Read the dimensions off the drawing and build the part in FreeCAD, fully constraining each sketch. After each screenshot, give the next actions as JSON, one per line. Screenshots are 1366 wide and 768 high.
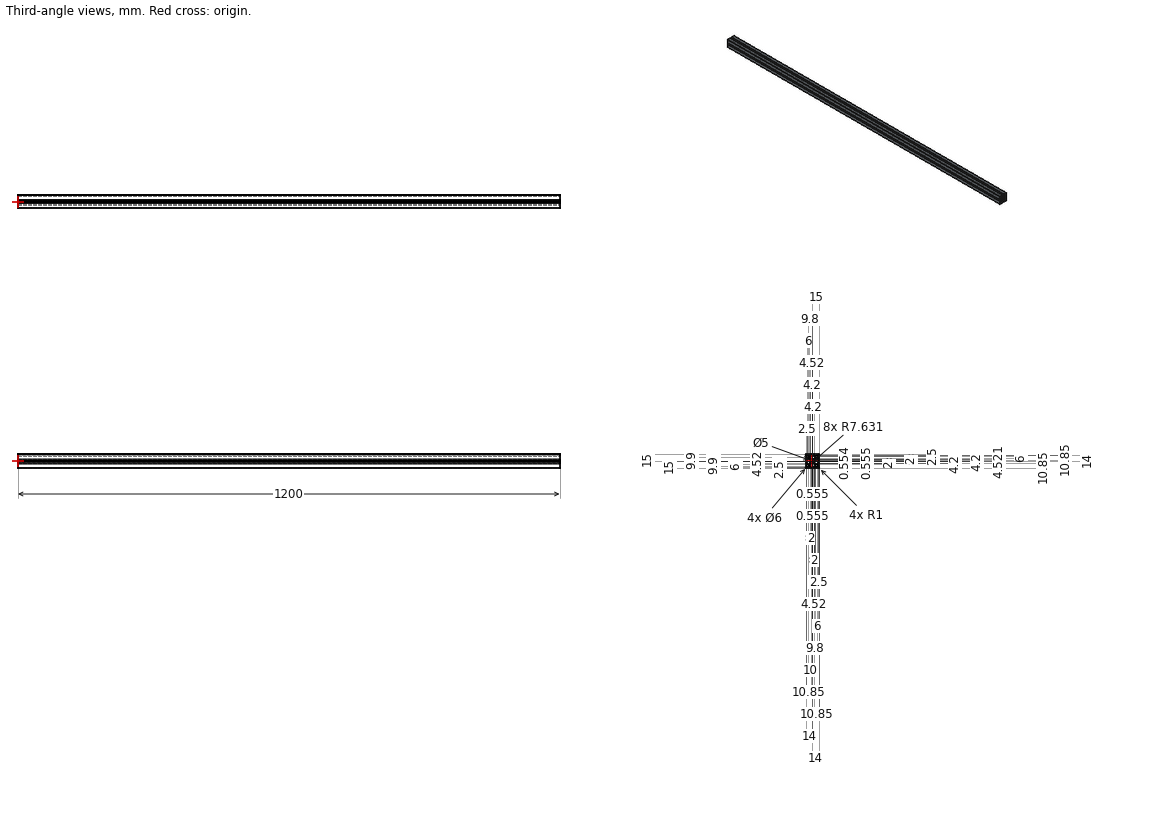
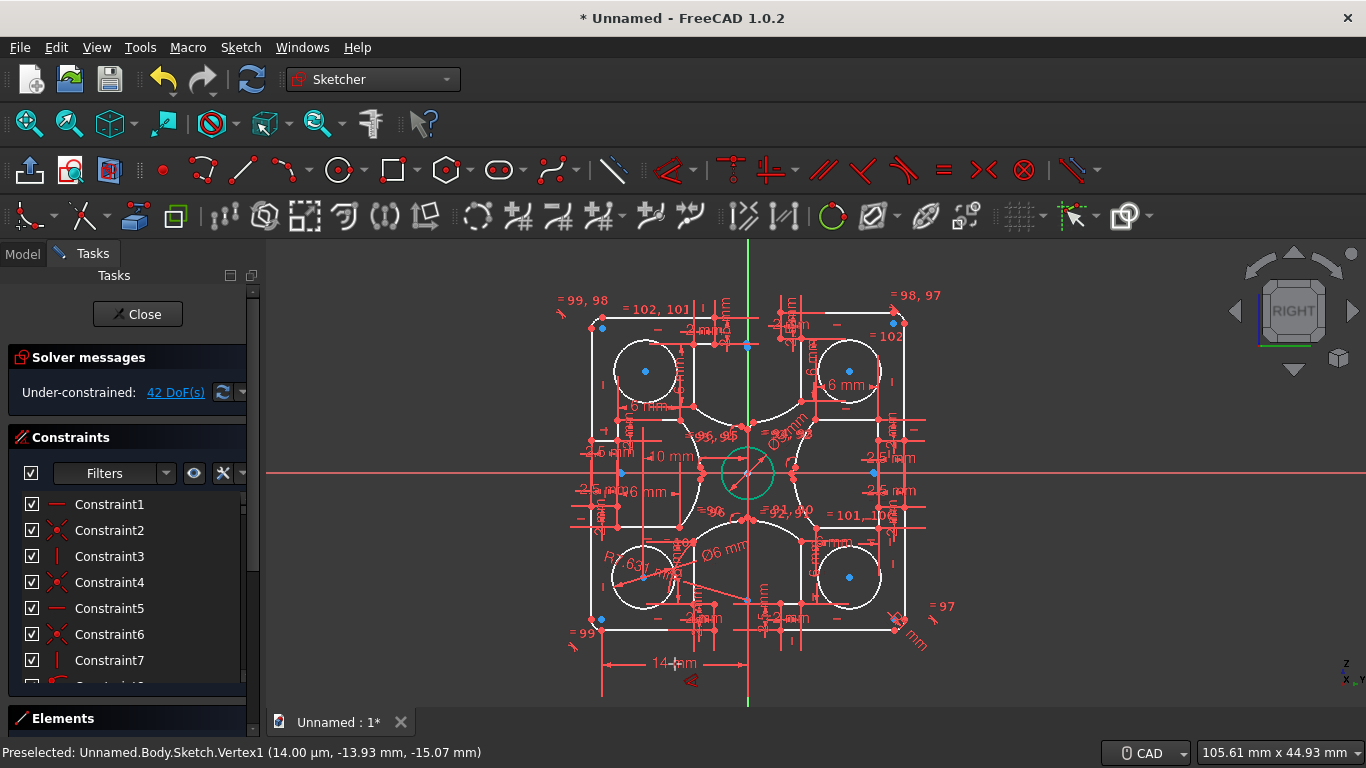
{"action": "left_click", "coordinate": [602, 630]}
{"action": "left_click", "coordinate": [568, 552]}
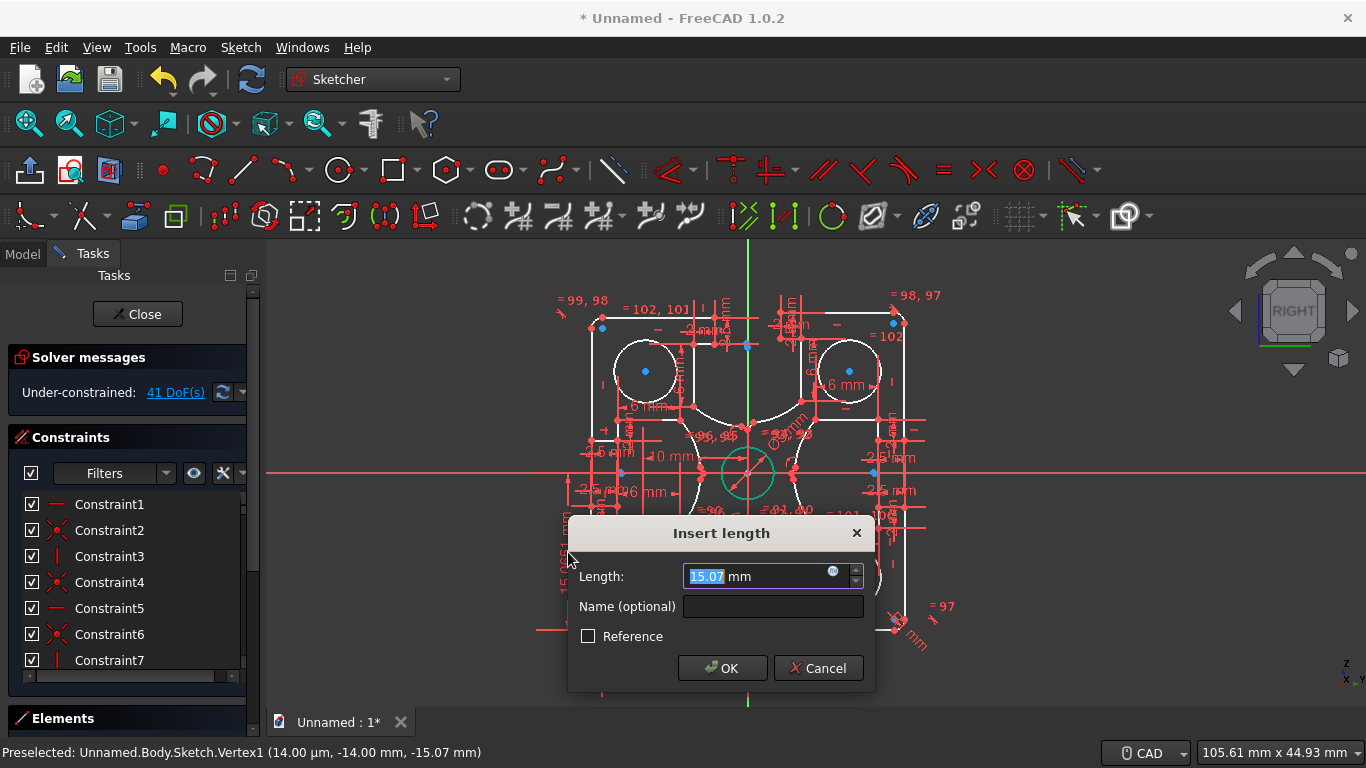
{"action": "type", "text": "15"}
{"action": "key", "text": "Return"}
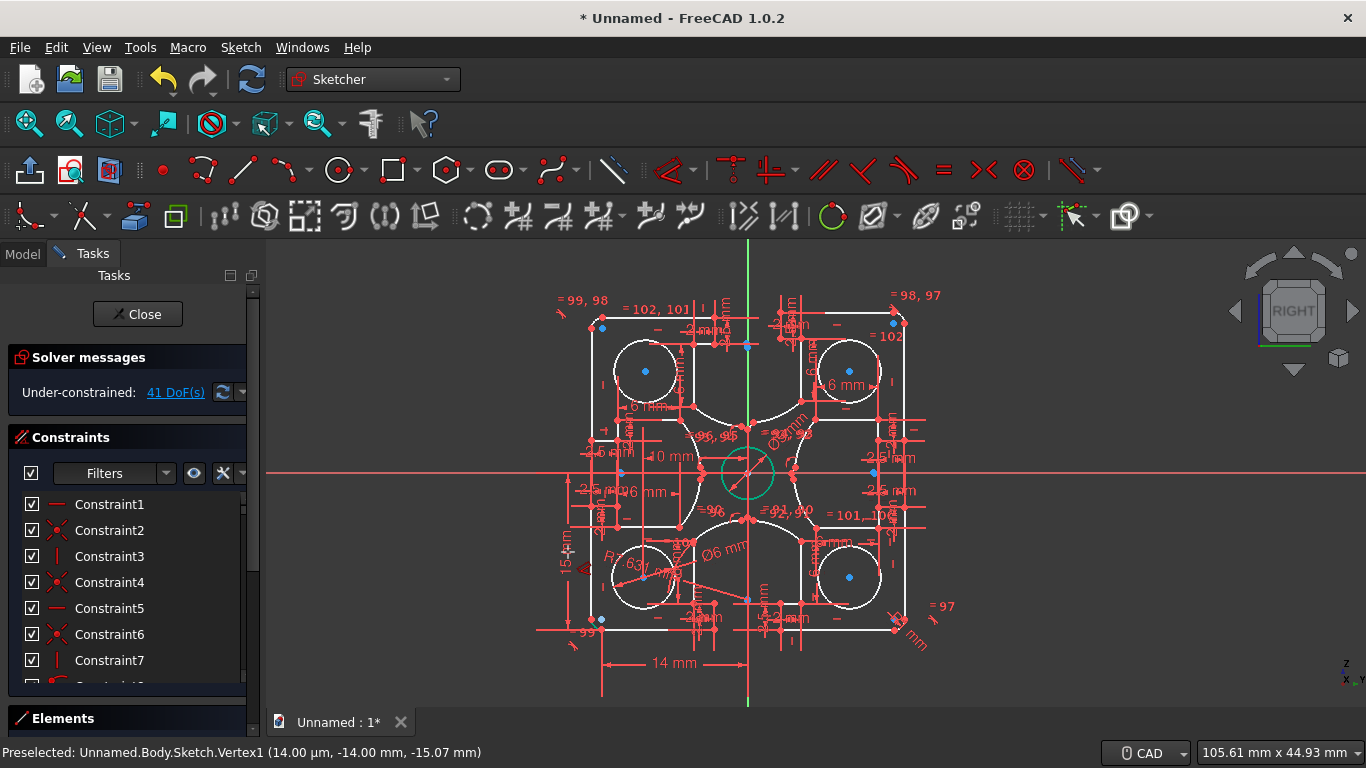
{"action": "left_click", "coordinate": [781, 630]}
{"action": "left_click", "coordinate": [815, 497]}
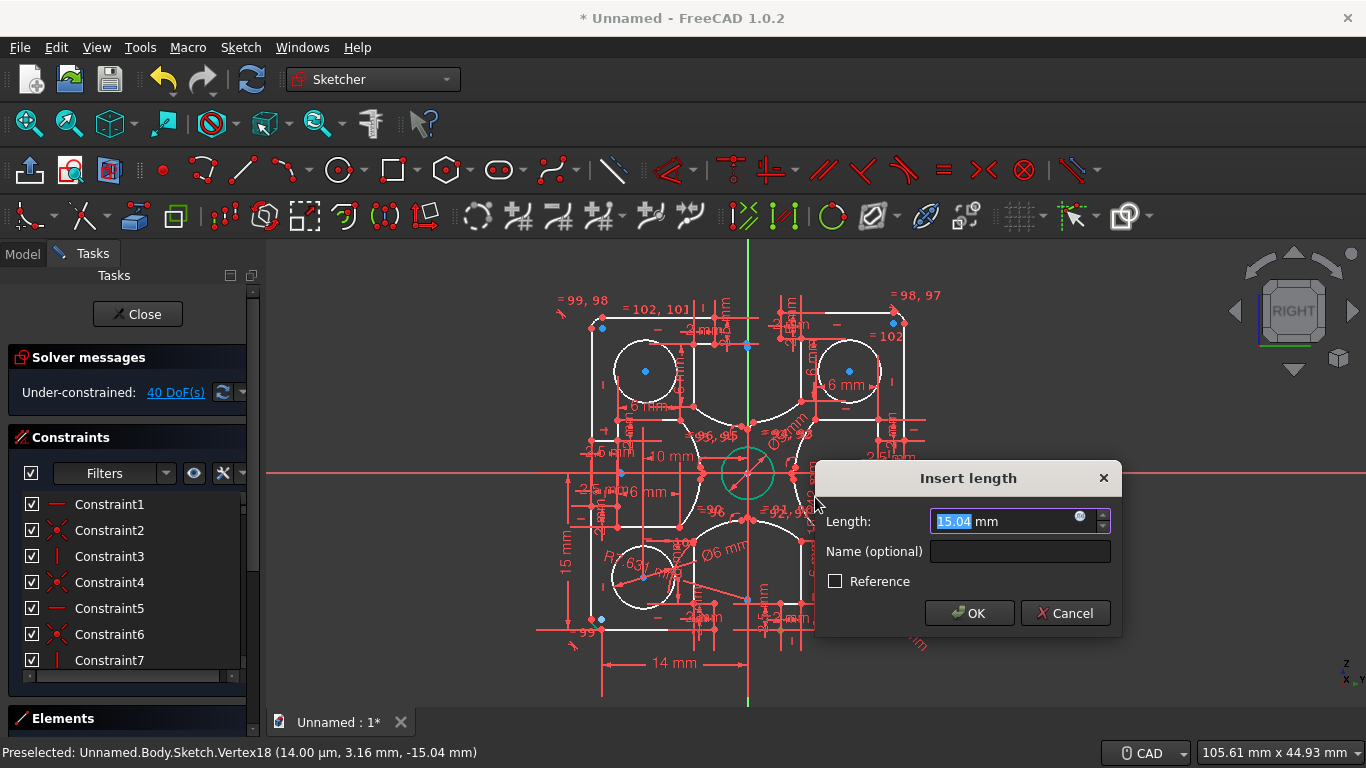
{"action": "type", "text": "15"}
{"action": "key", "text": "Return"}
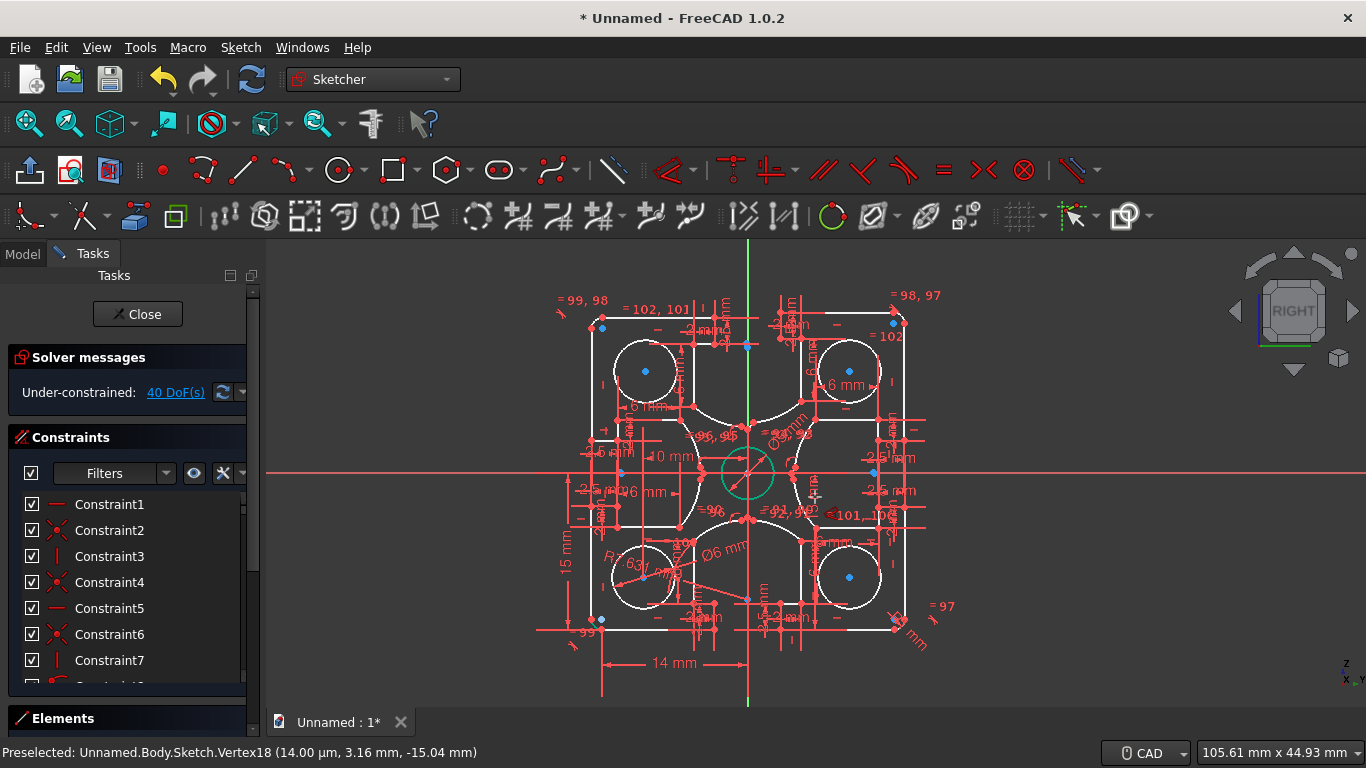
{"action": "left_click", "coordinate": [895, 630]}
{"action": "left_click", "coordinate": [821, 664]}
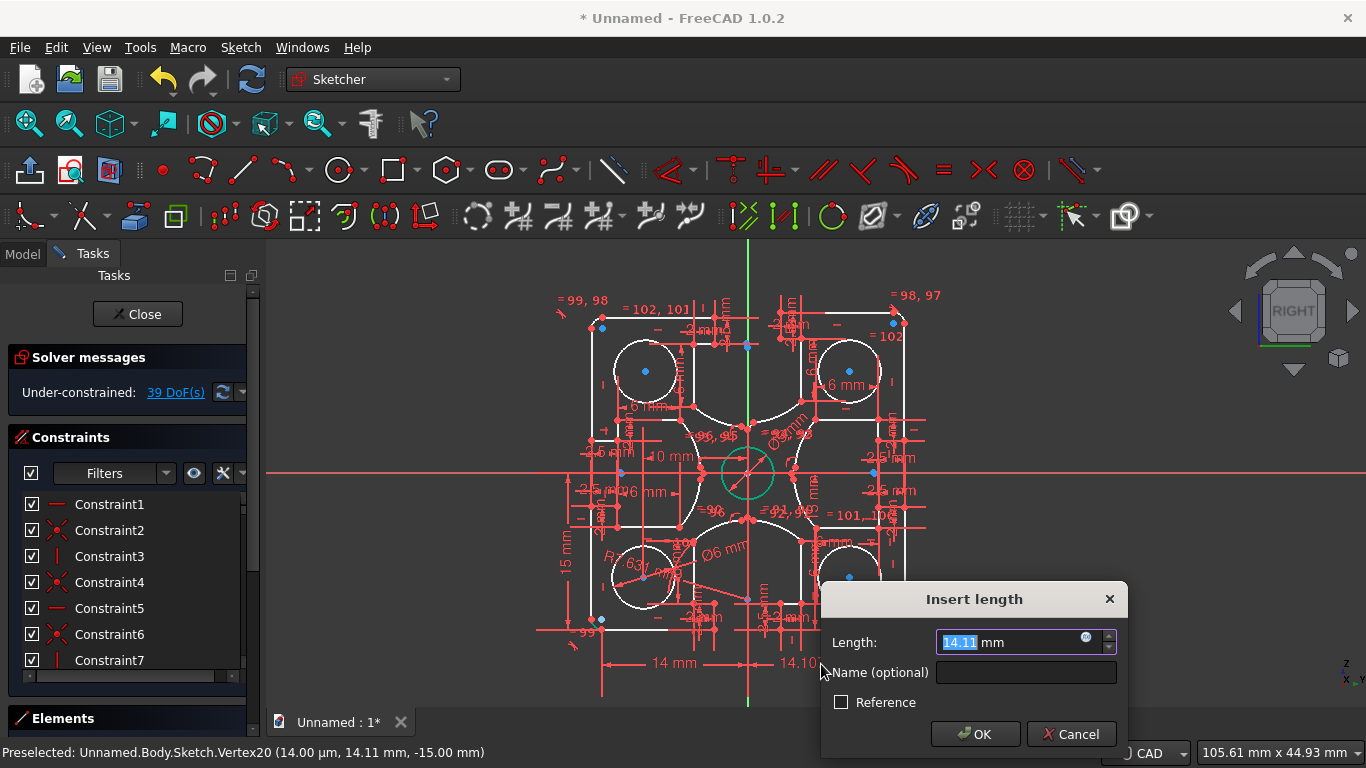
{"action": "type", "text": "14"}
{"action": "key", "text": "Return"}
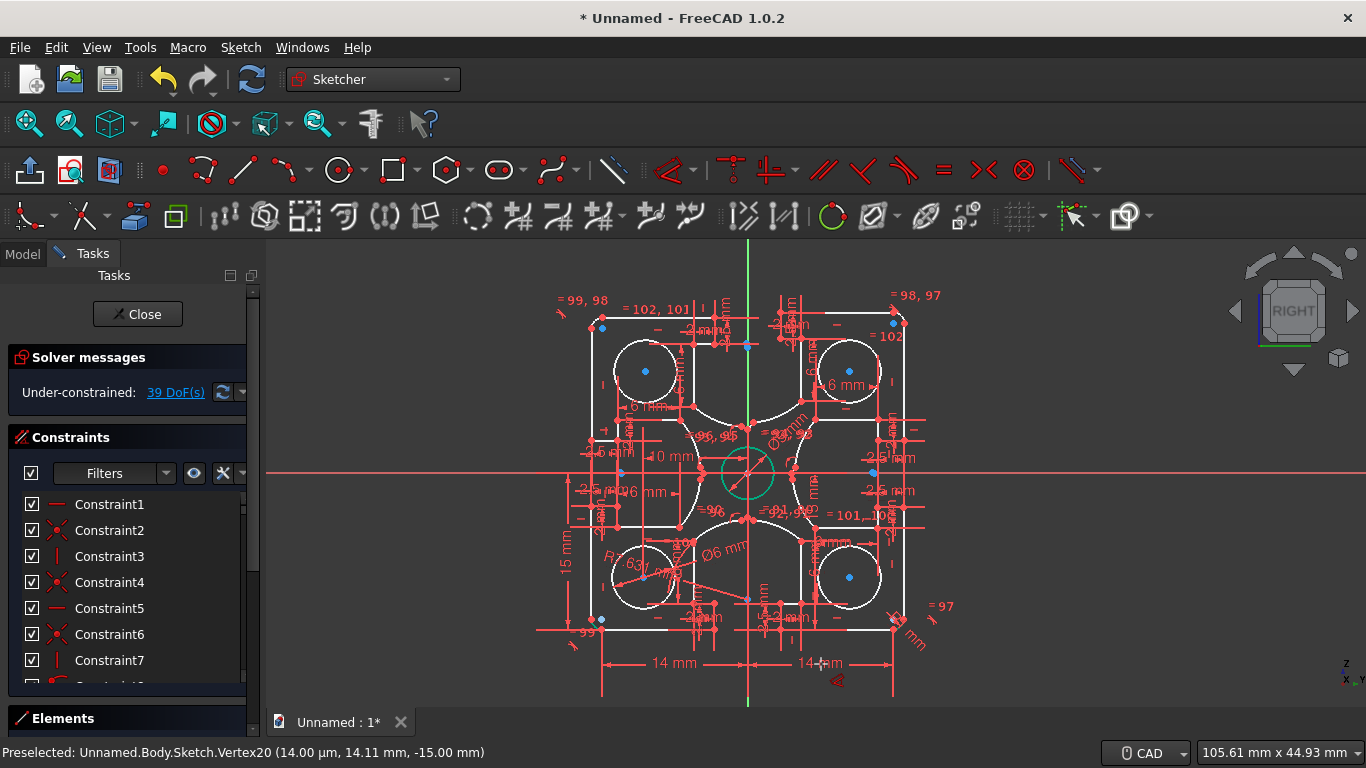
{"action": "left_click", "coordinate": [904, 441]}
{"action": "left_click", "coordinate": [881, 407]}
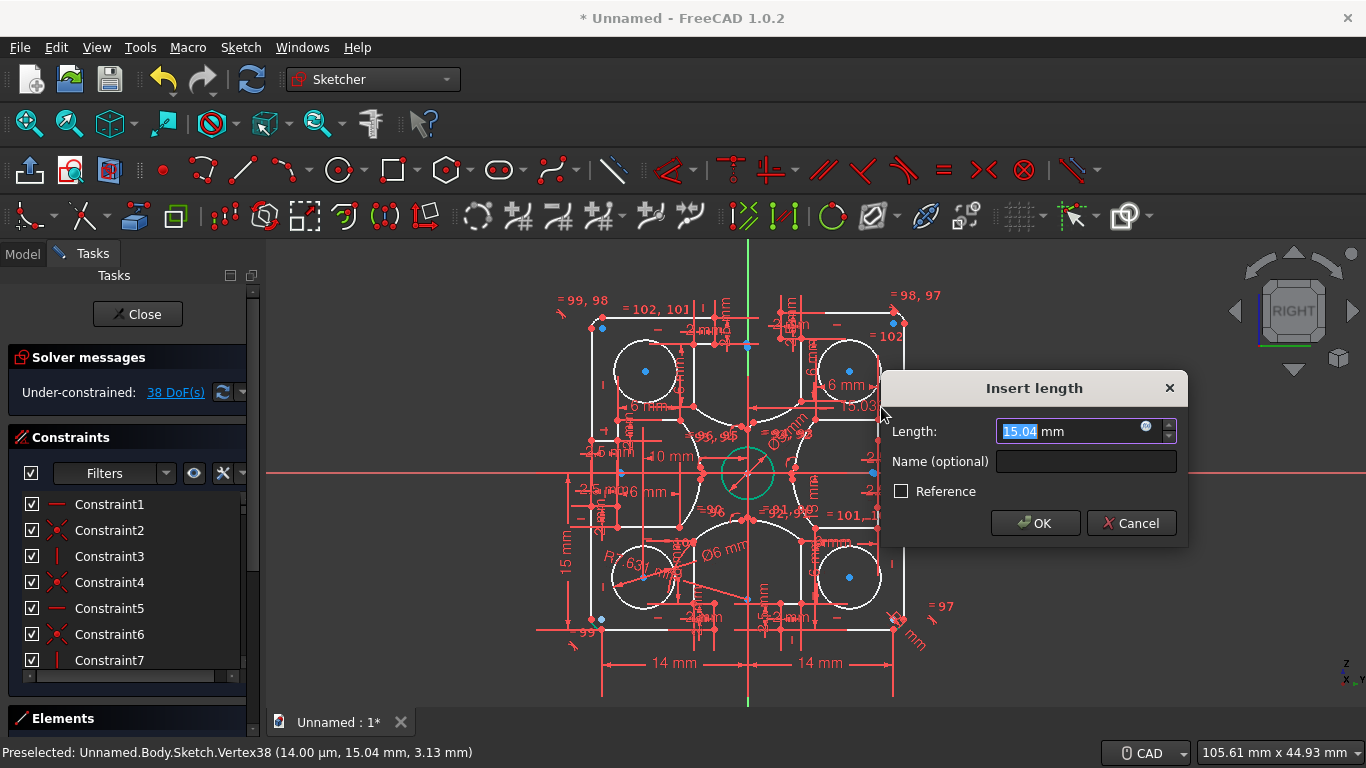
{"action": "type", "text": "15"}
{"action": "key", "text": "Return"}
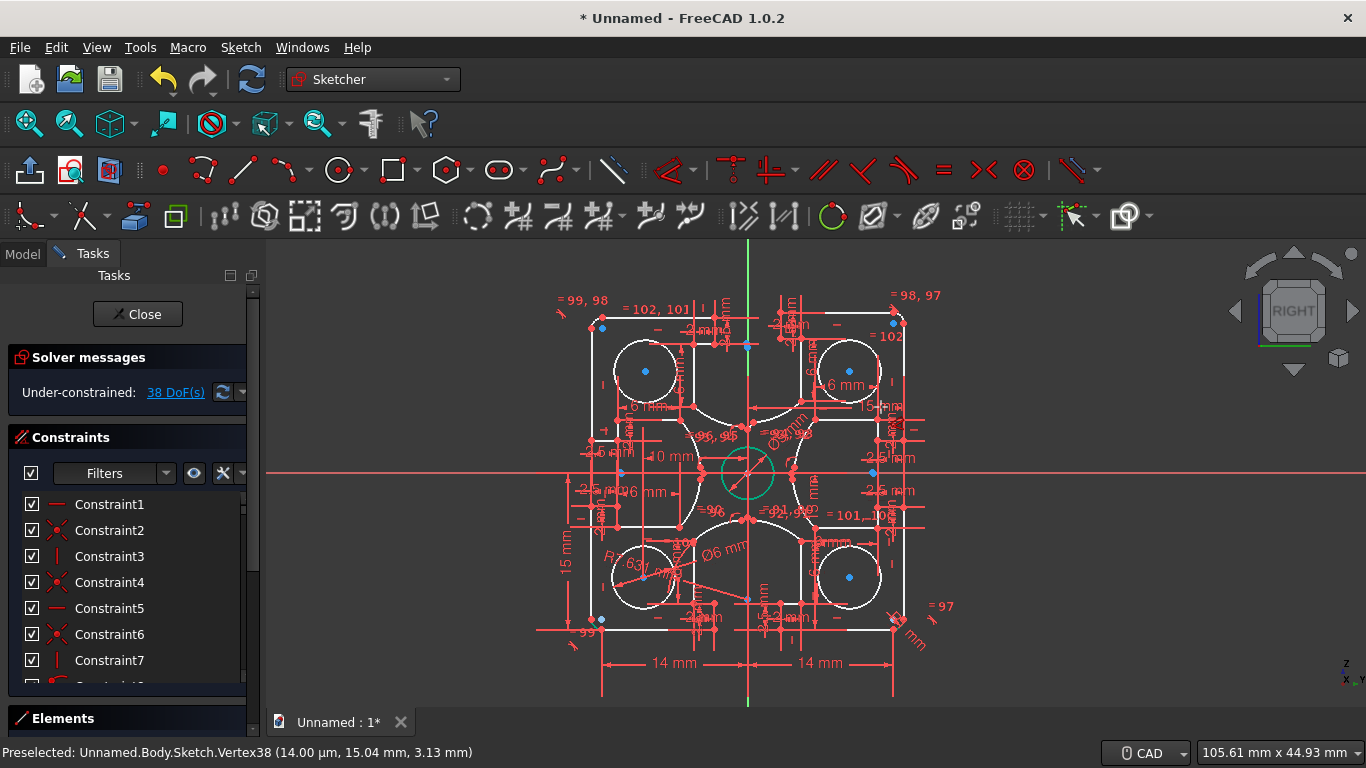
{"action": "left_click", "coordinate": [904, 323]}
{"action": "left_click", "coordinate": [938, 364]}